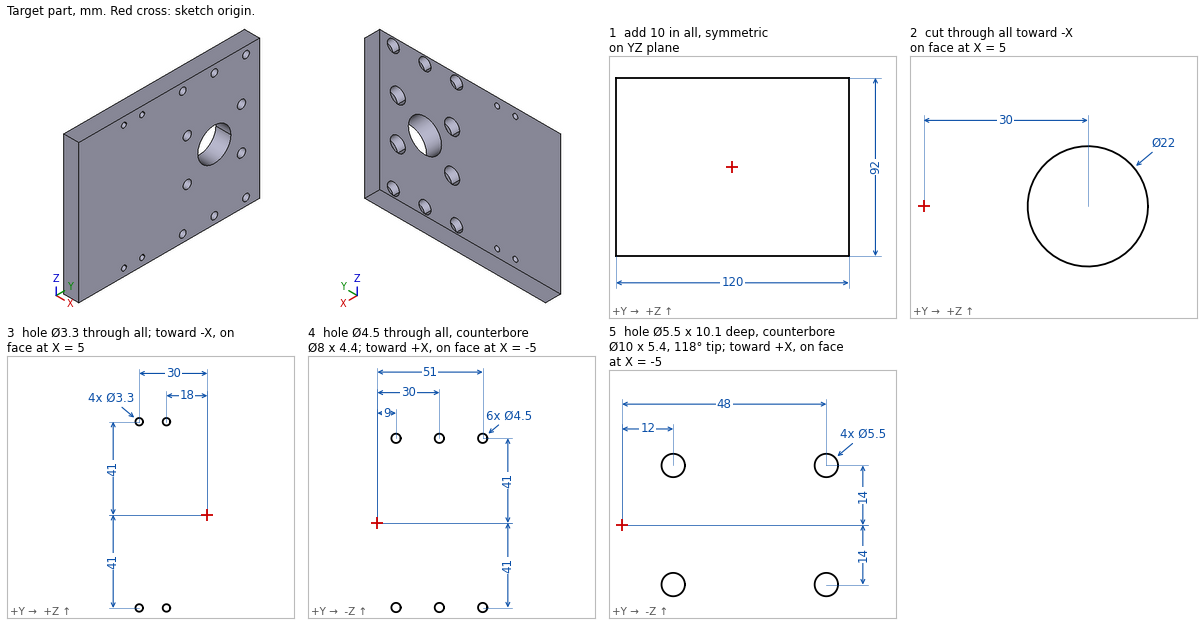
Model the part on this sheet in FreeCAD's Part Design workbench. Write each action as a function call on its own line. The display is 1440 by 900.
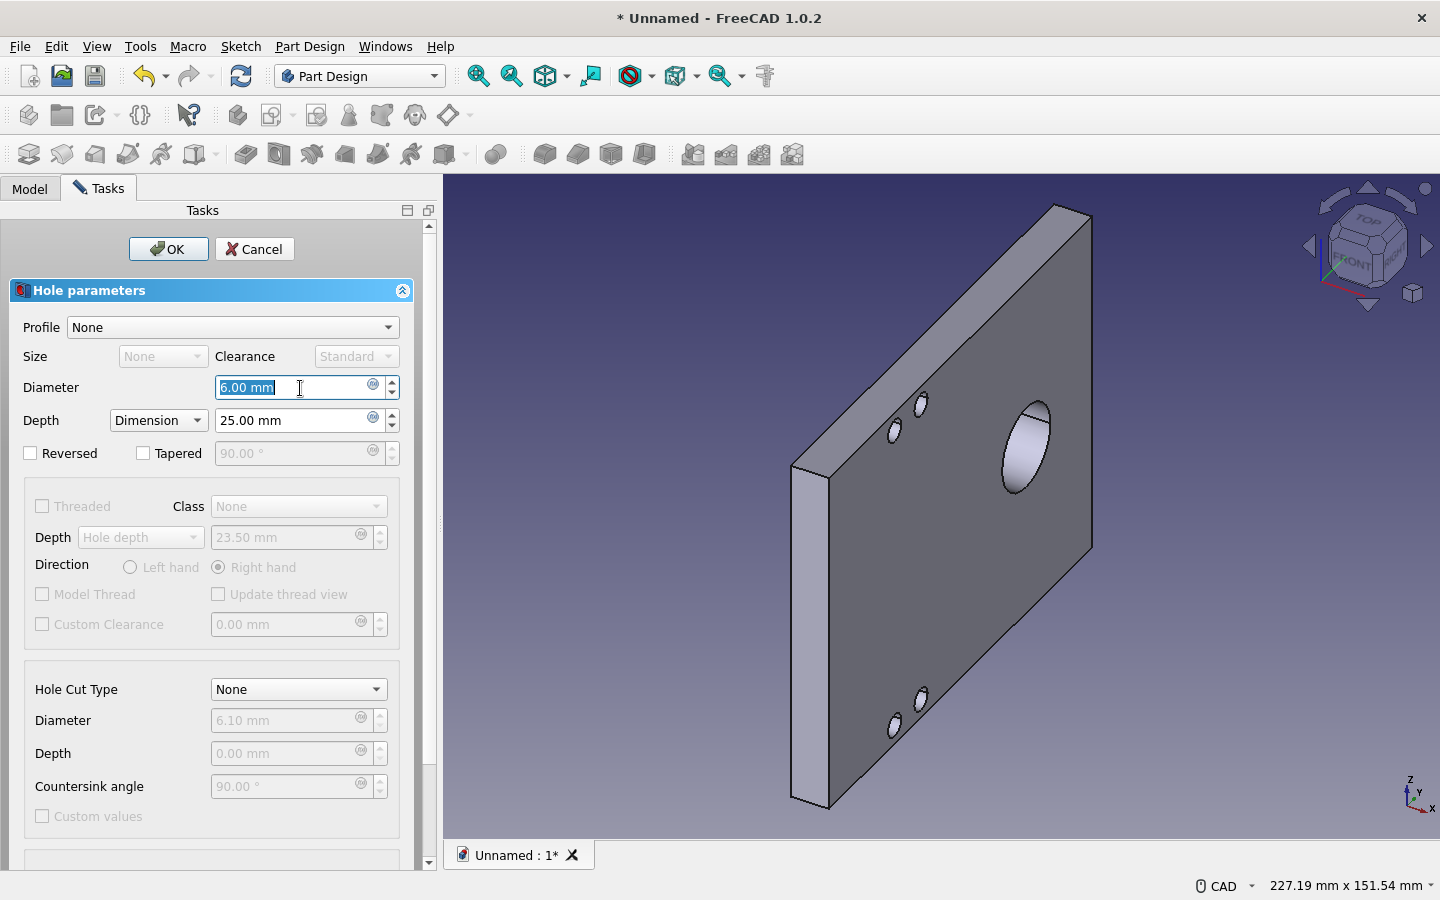
text(3.3)
key(Tab)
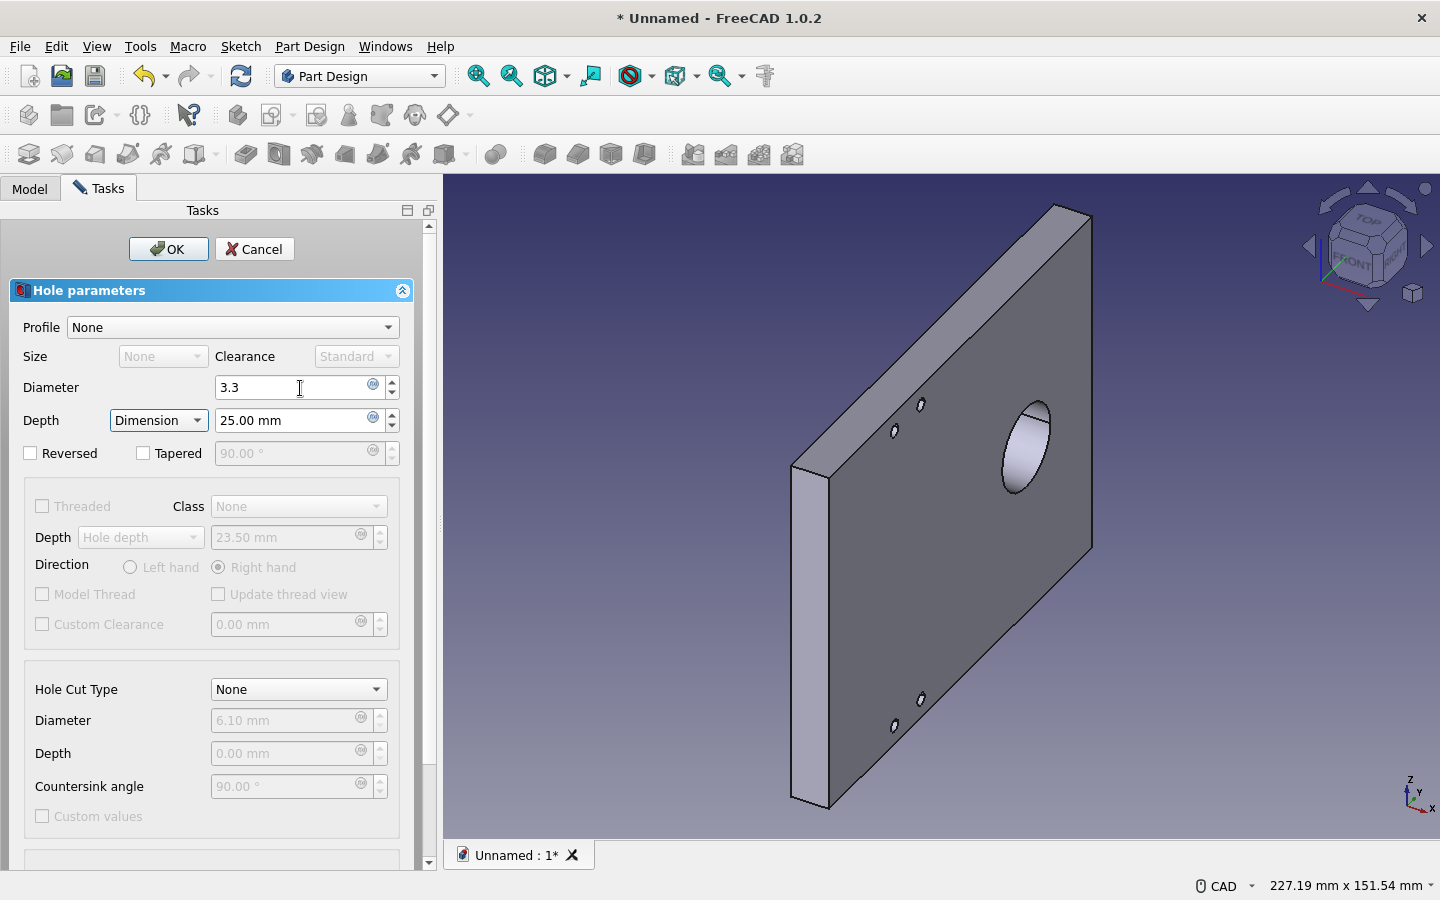
click(160, 420)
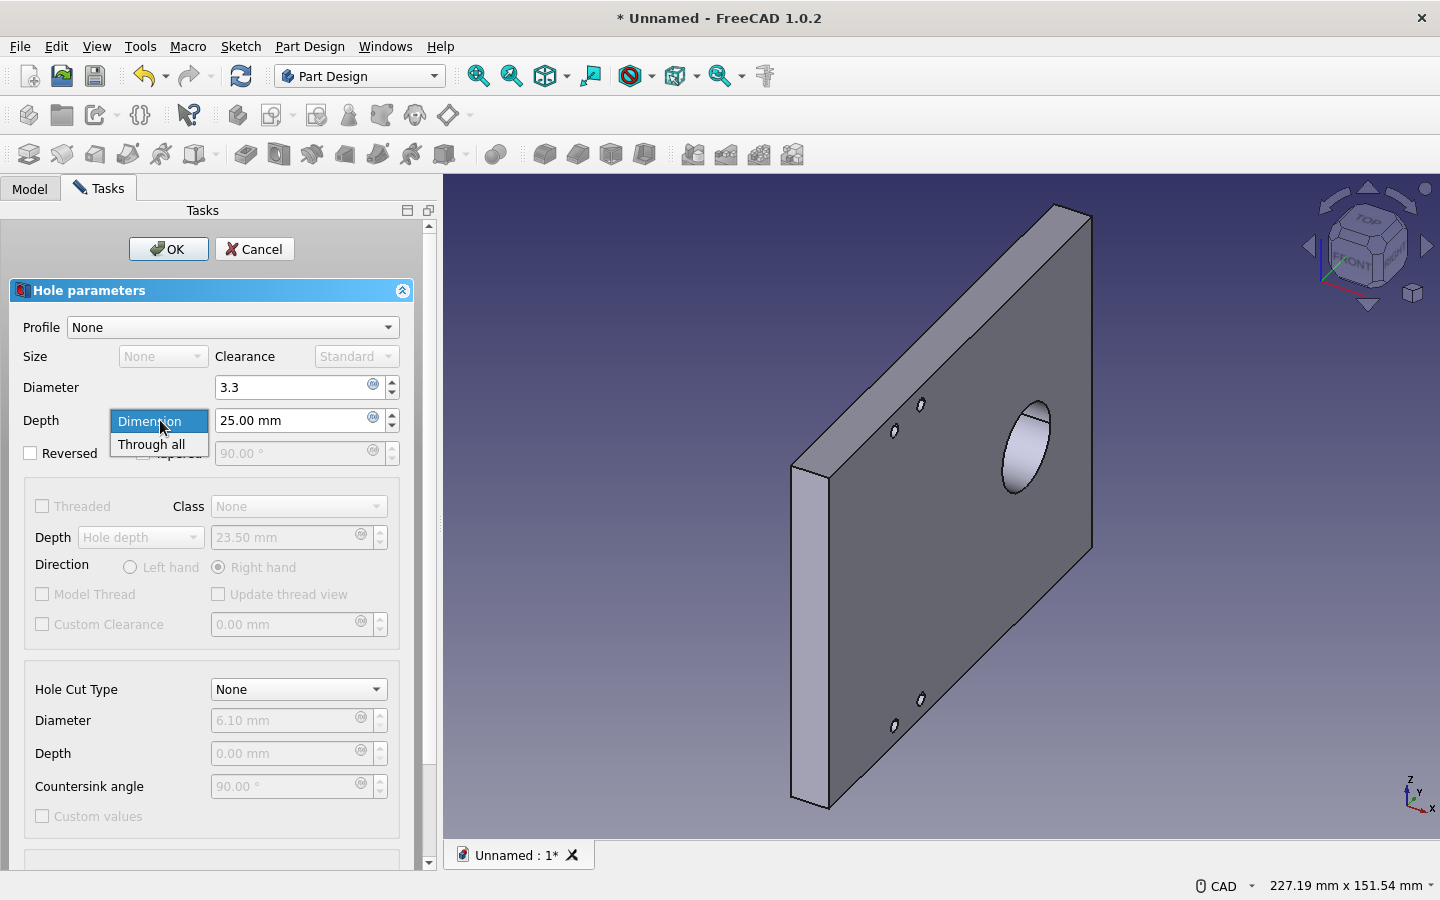
click(158, 444)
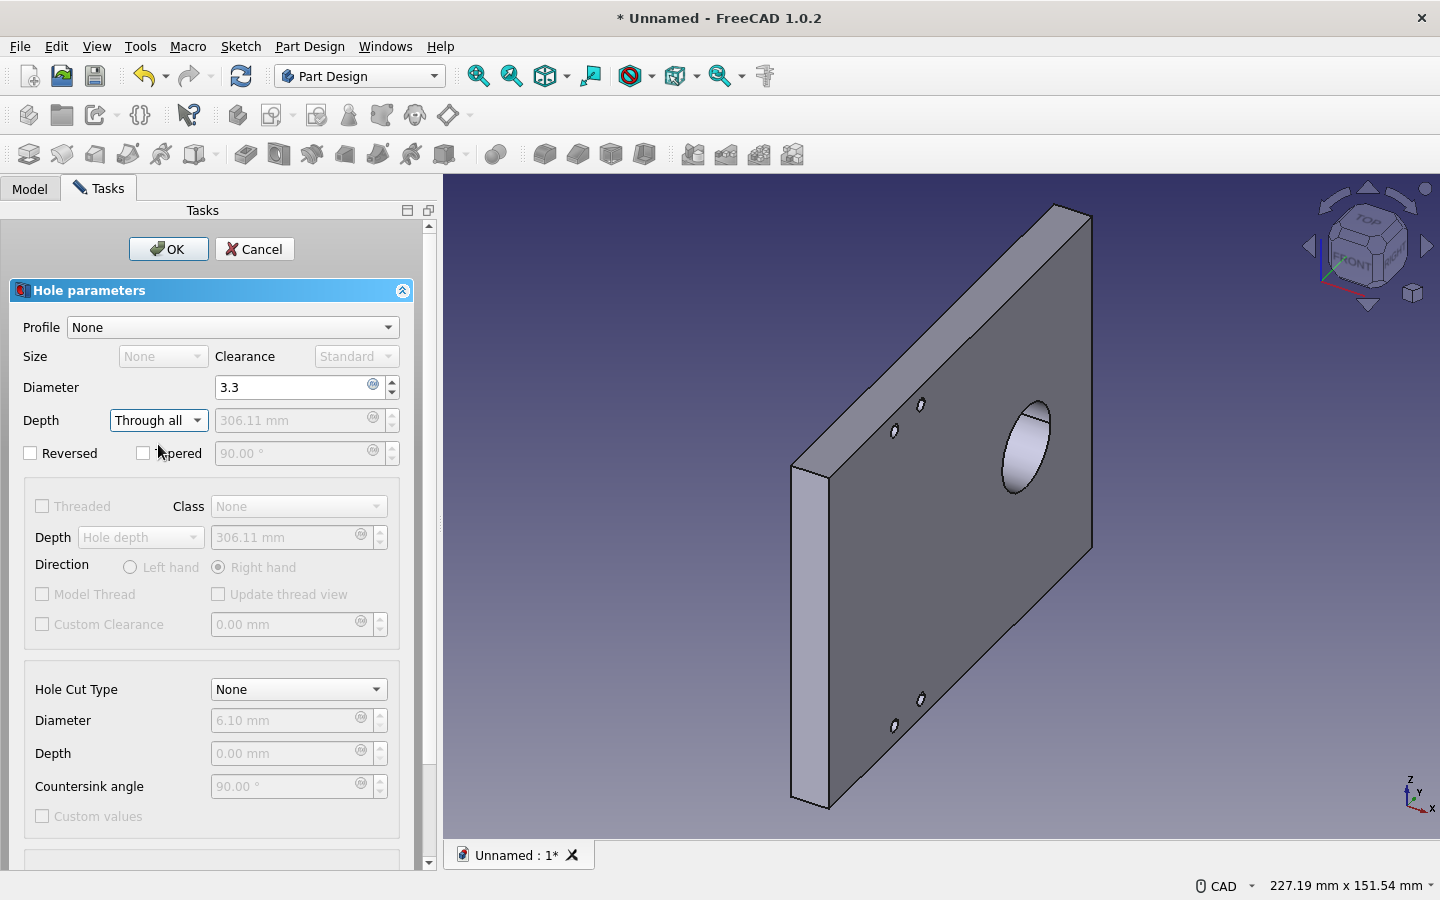
click(169, 249)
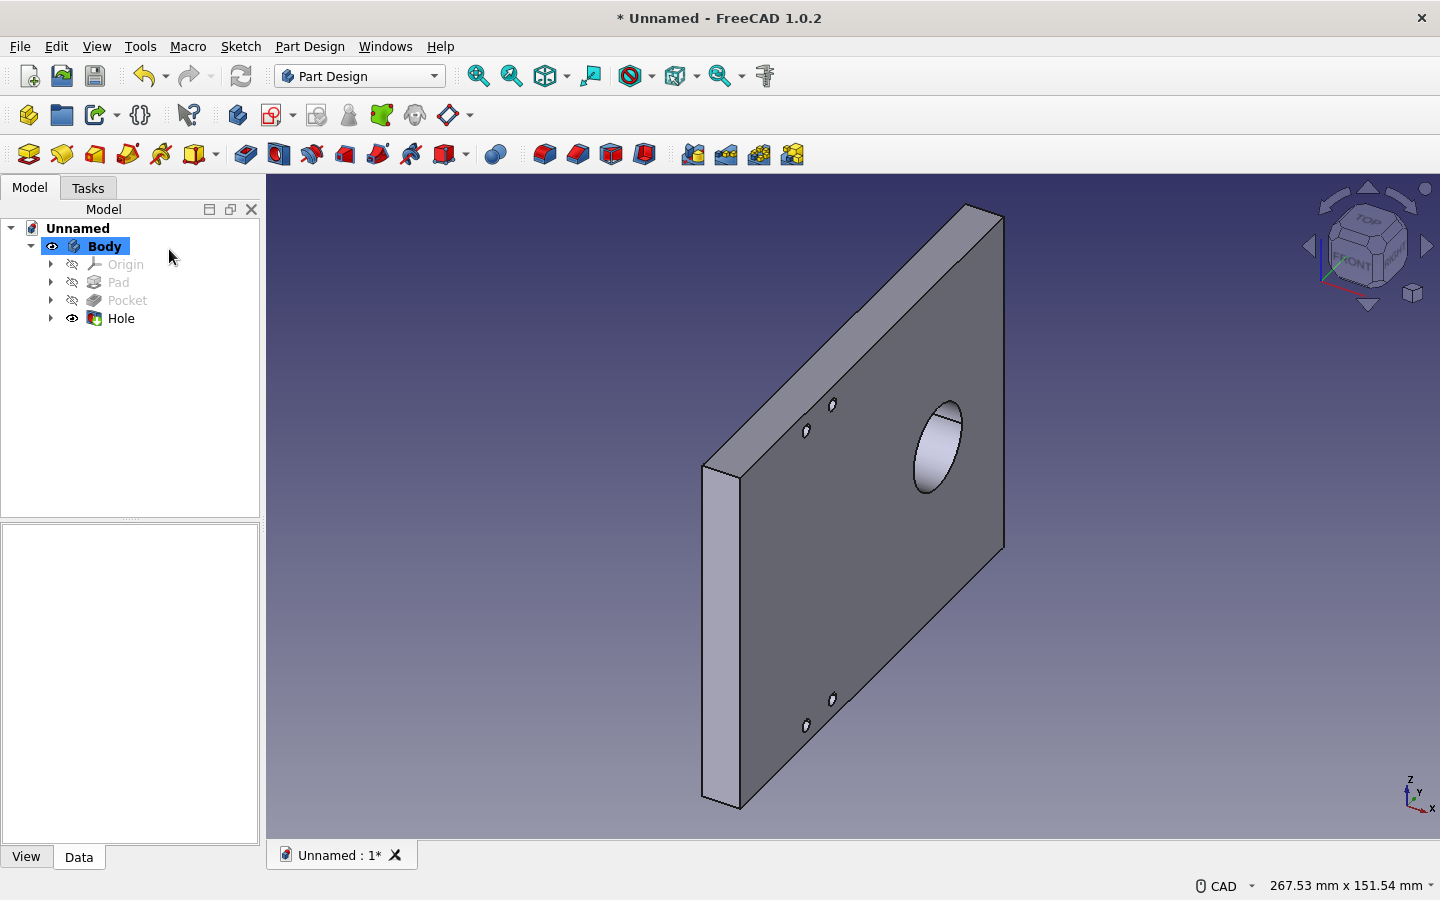
key(6)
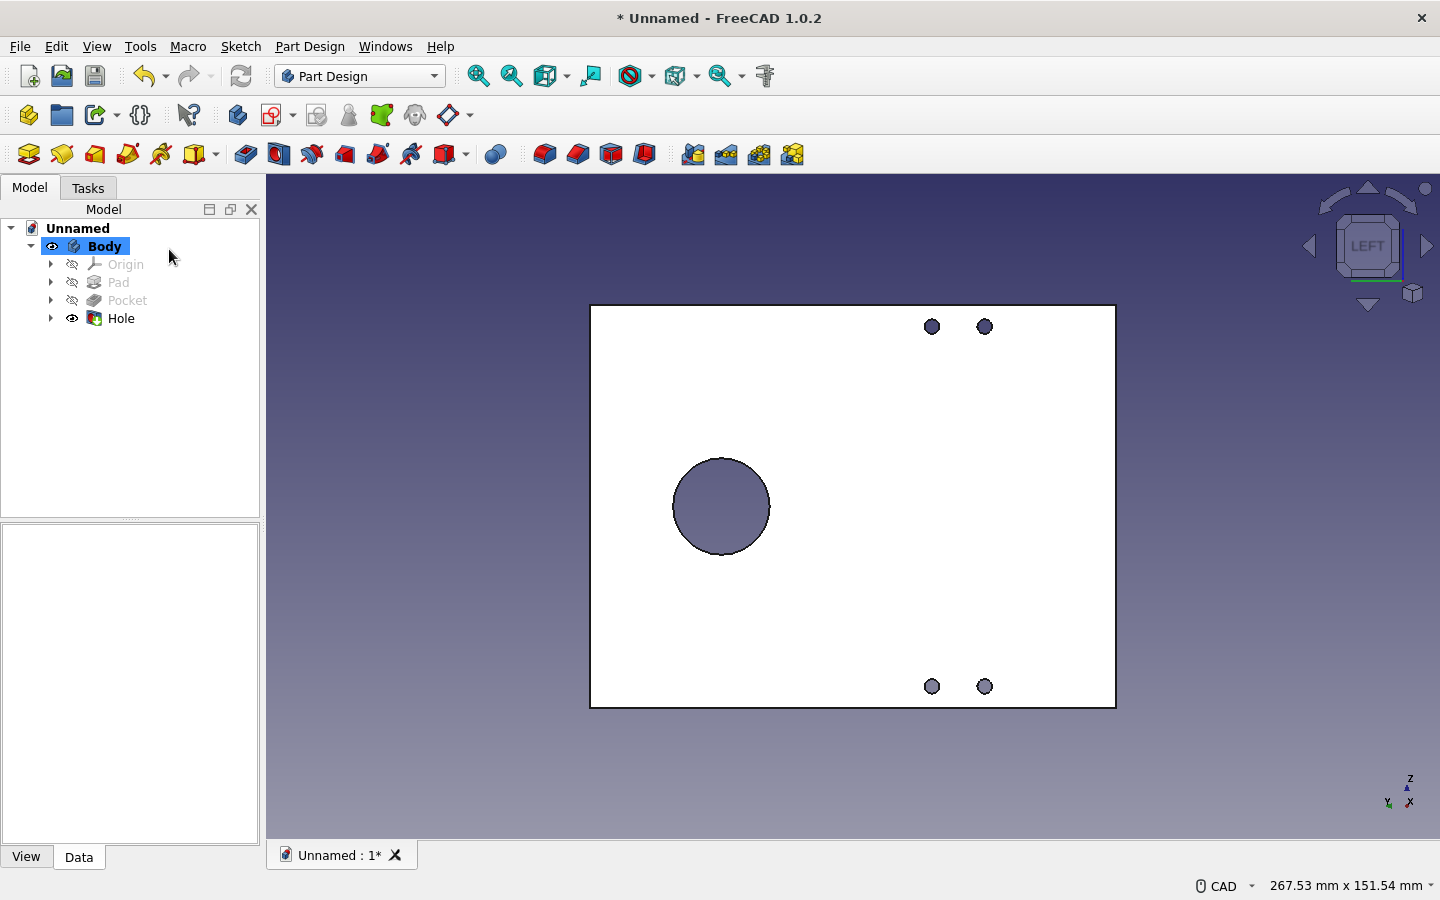
click(928, 505)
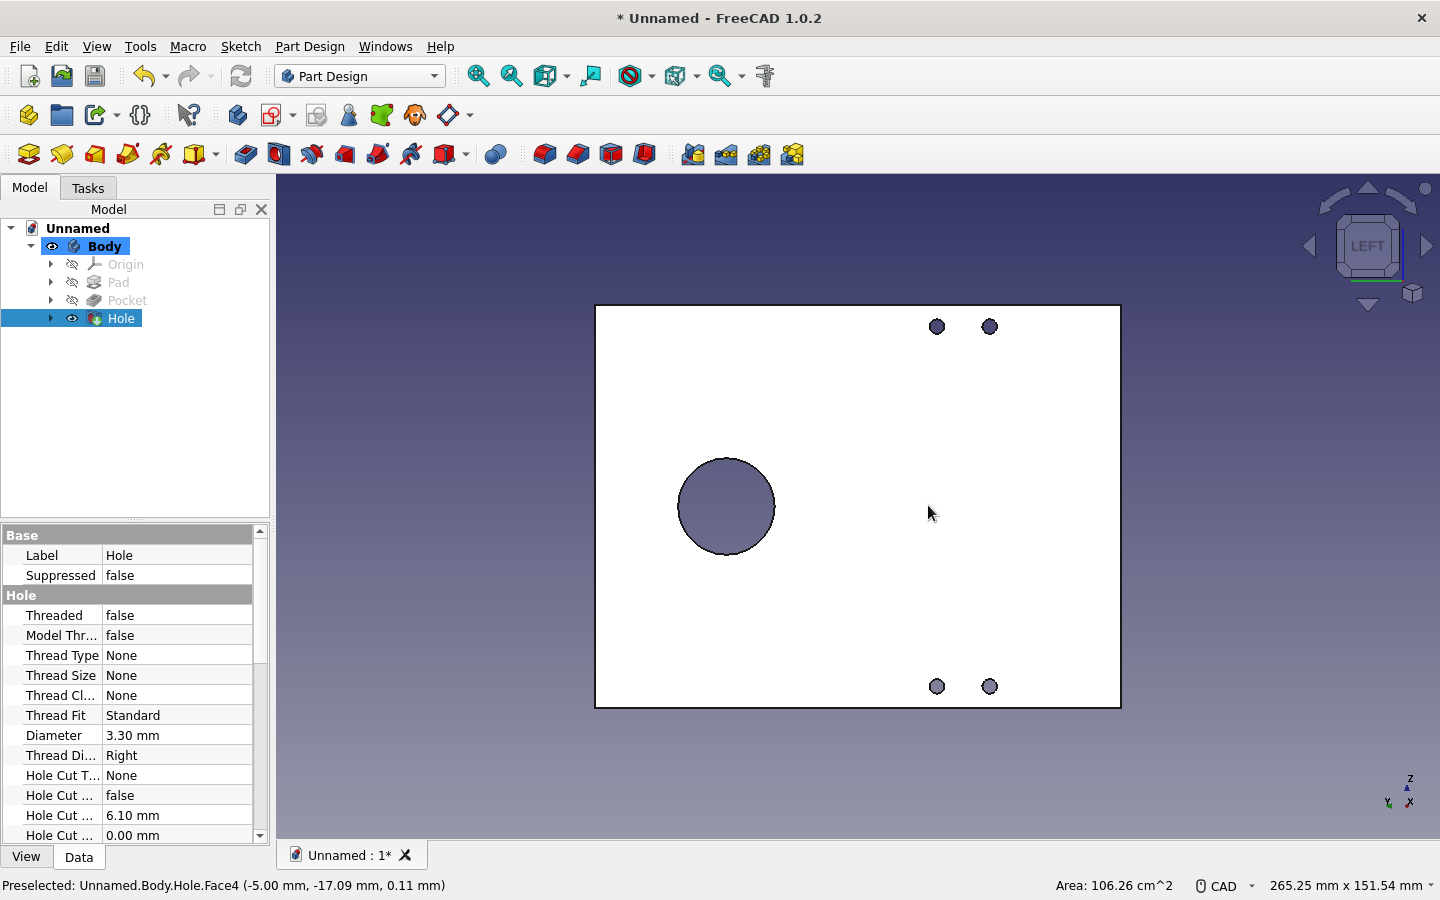
click(270, 116)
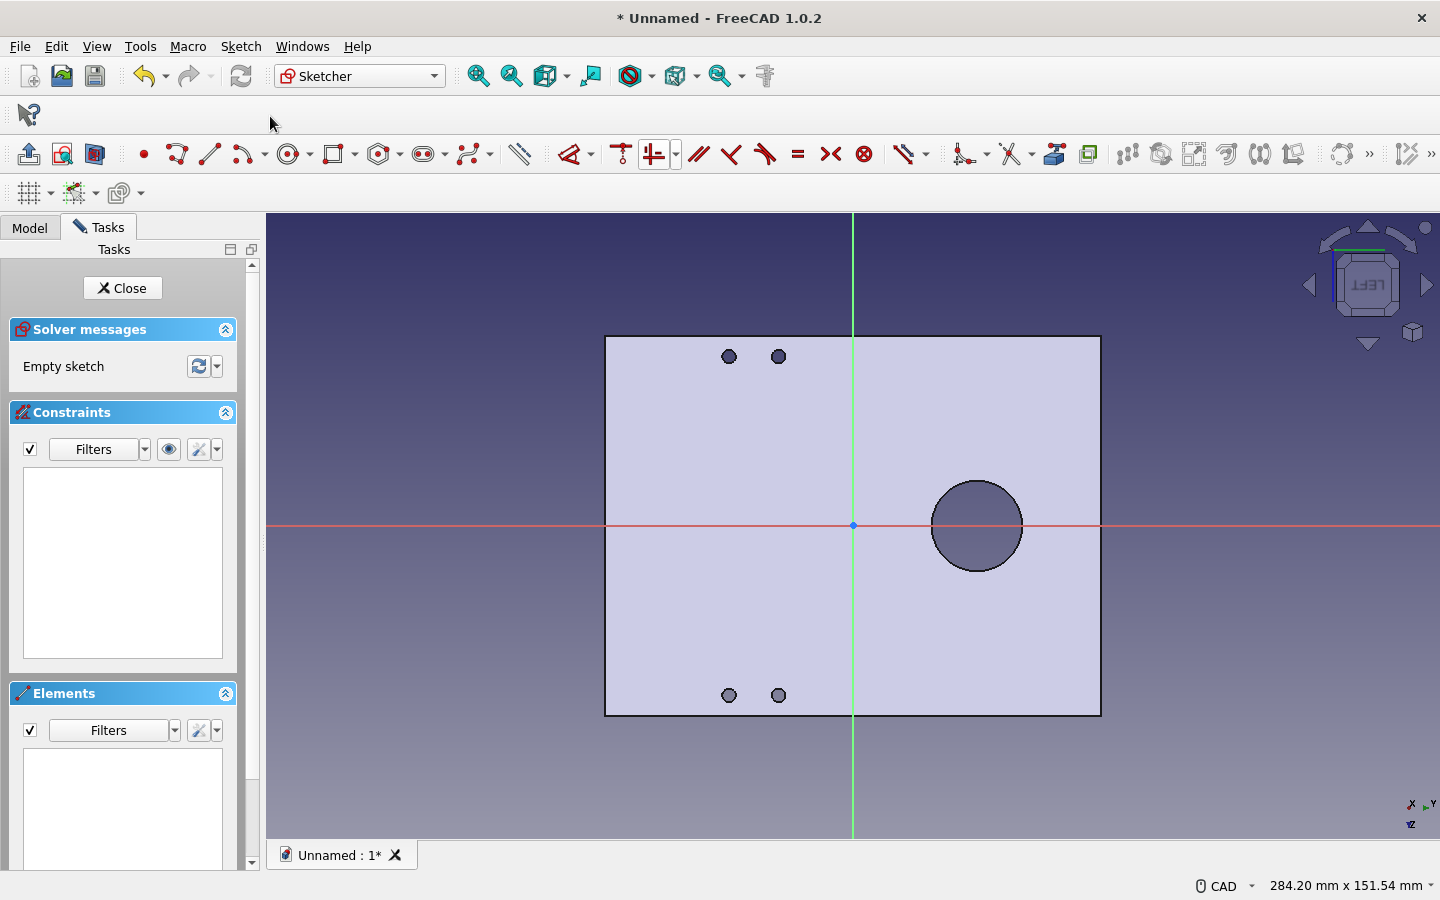
key(g)
key(c)